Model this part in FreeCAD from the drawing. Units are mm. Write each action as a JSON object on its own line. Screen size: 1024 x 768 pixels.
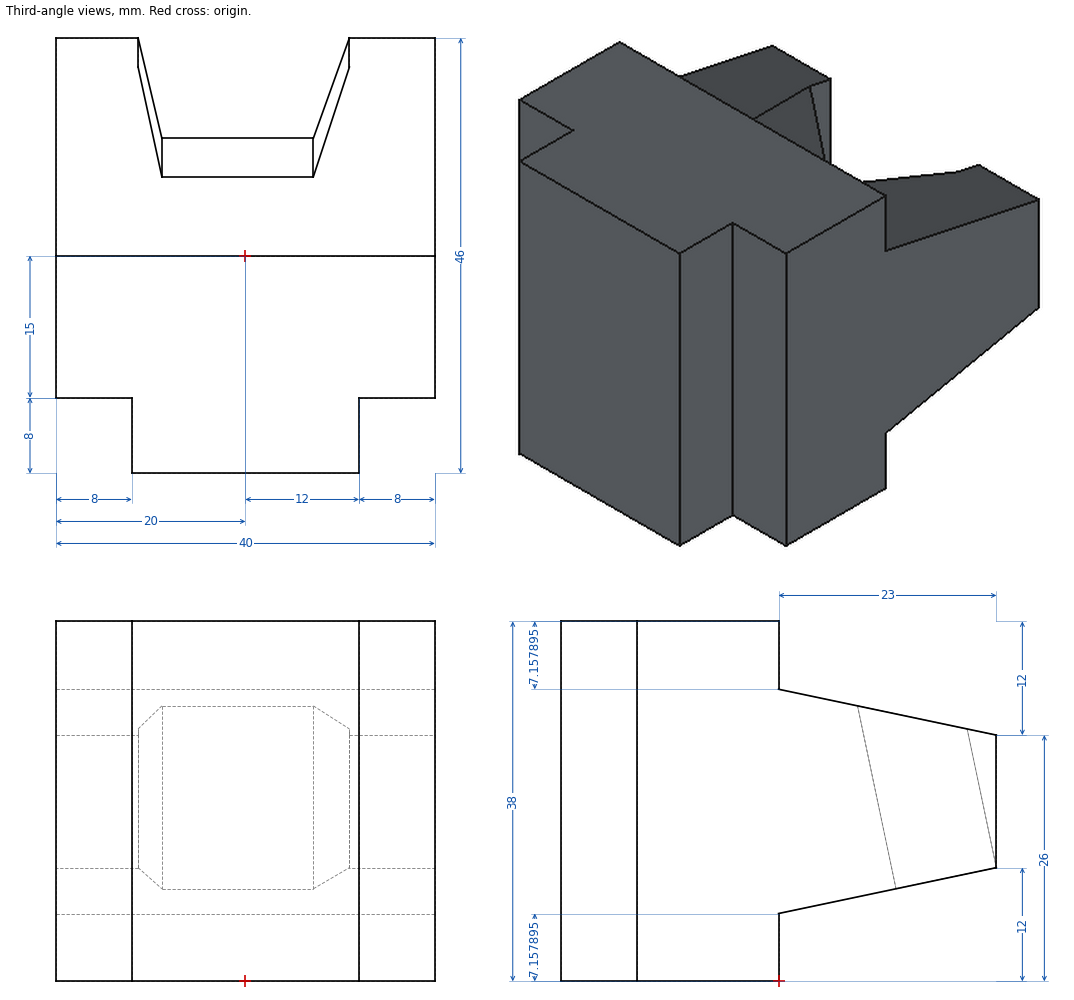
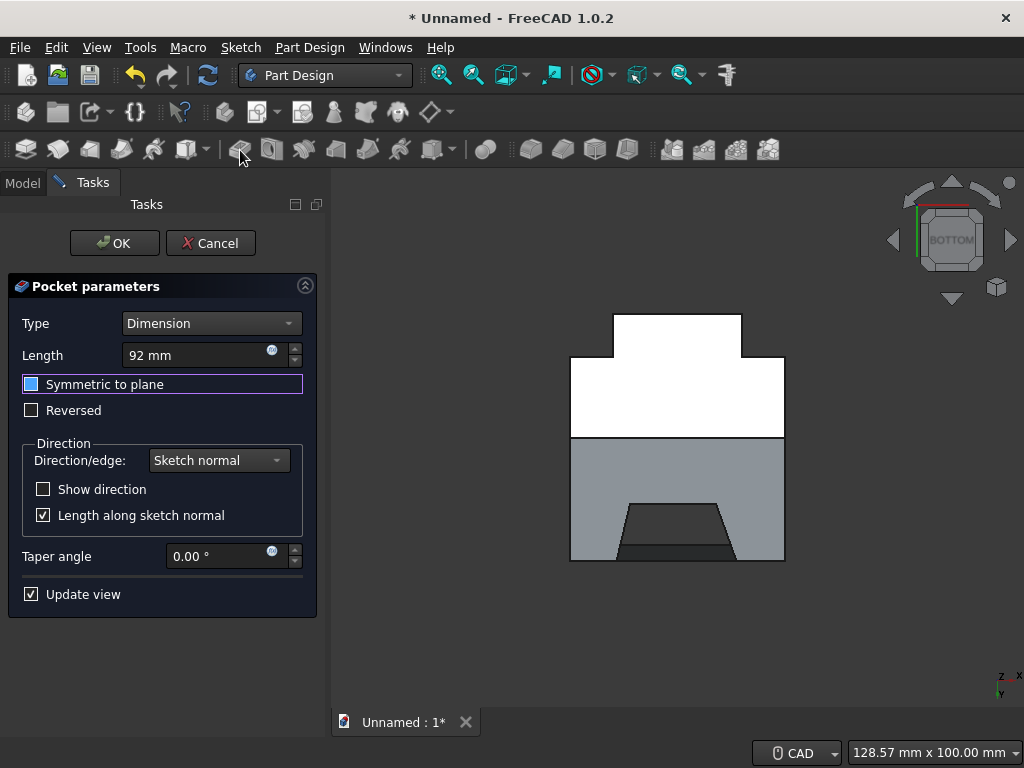
{"action": "left_click", "coordinate": [30, 384]}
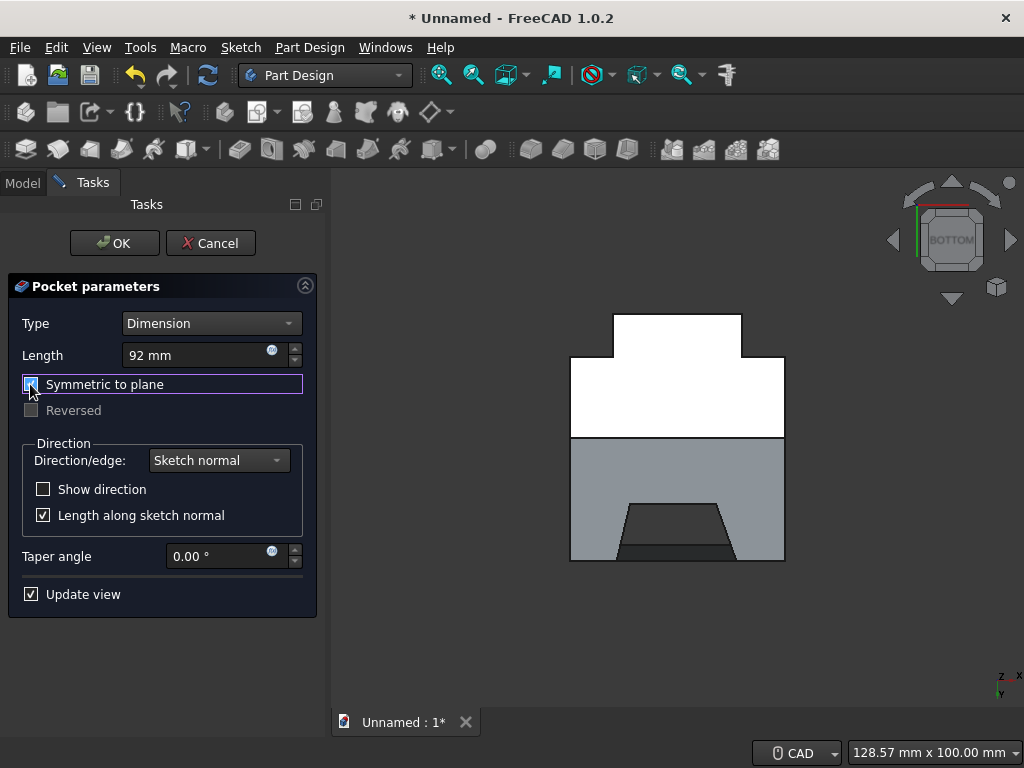
{"action": "left_click", "coordinate": [115, 243]}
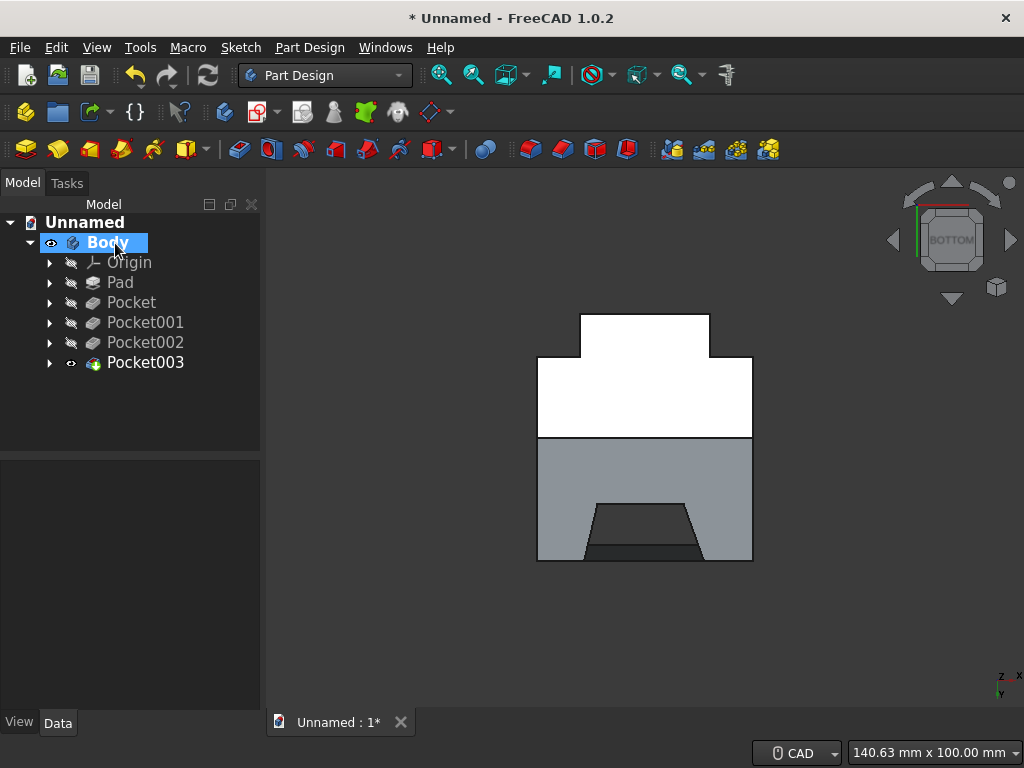
{"action": "left_click", "coordinate": [707, 481]}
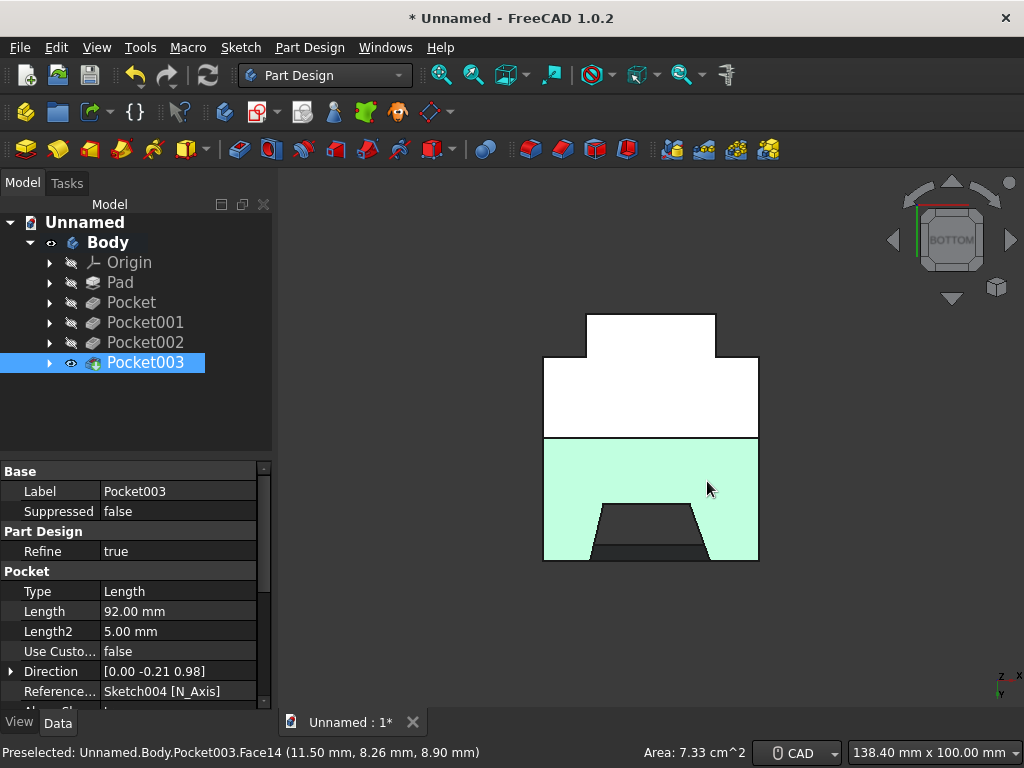
{"action": "left_click", "coordinate": [258, 112]}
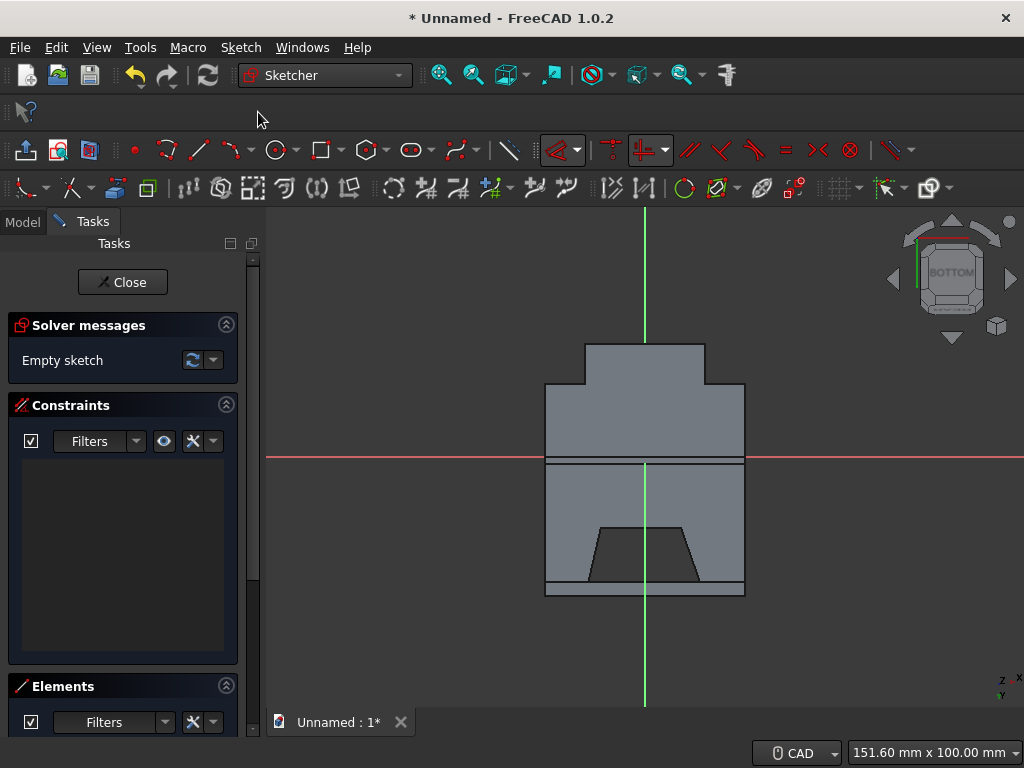
{"action": "left_click", "coordinate": [90, 150]}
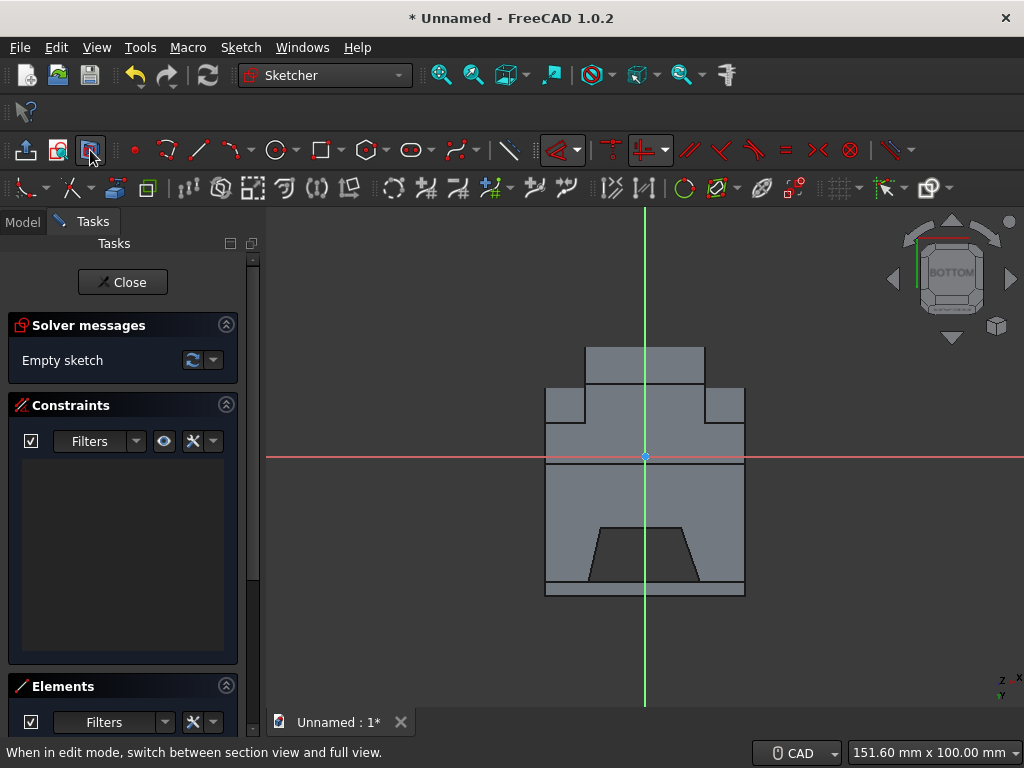
{"action": "scroll", "coordinate": [699, 592], "scroll_direction": "up", "scroll_amount": 4}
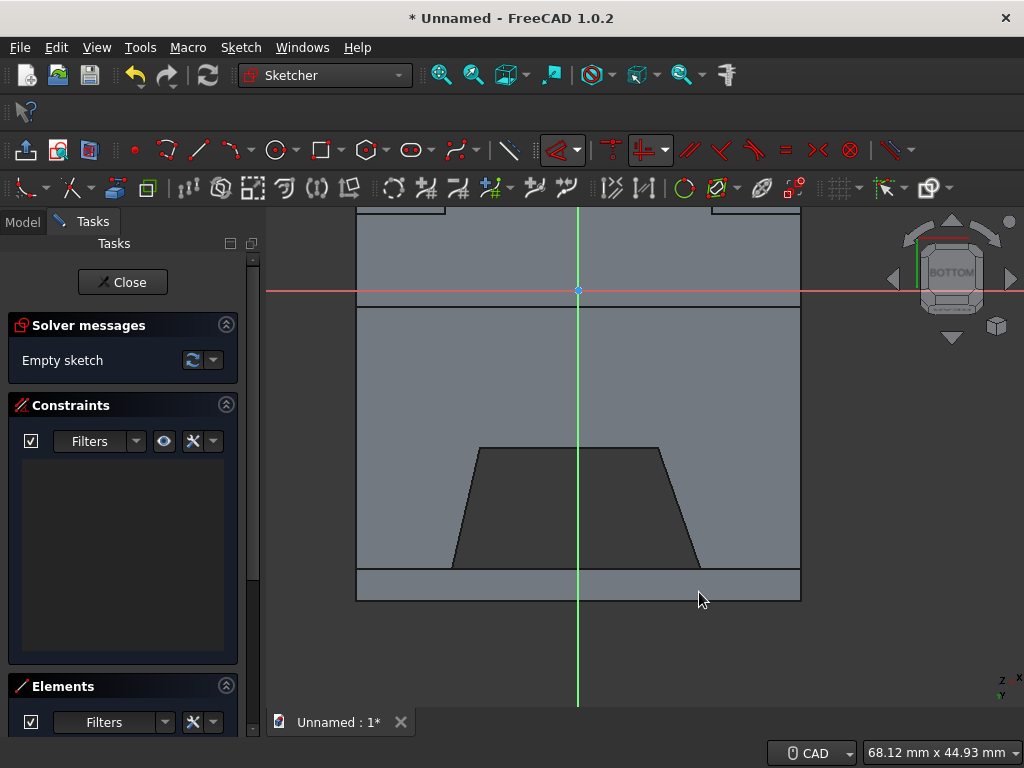
{"action": "left_click", "coordinate": [322, 150]}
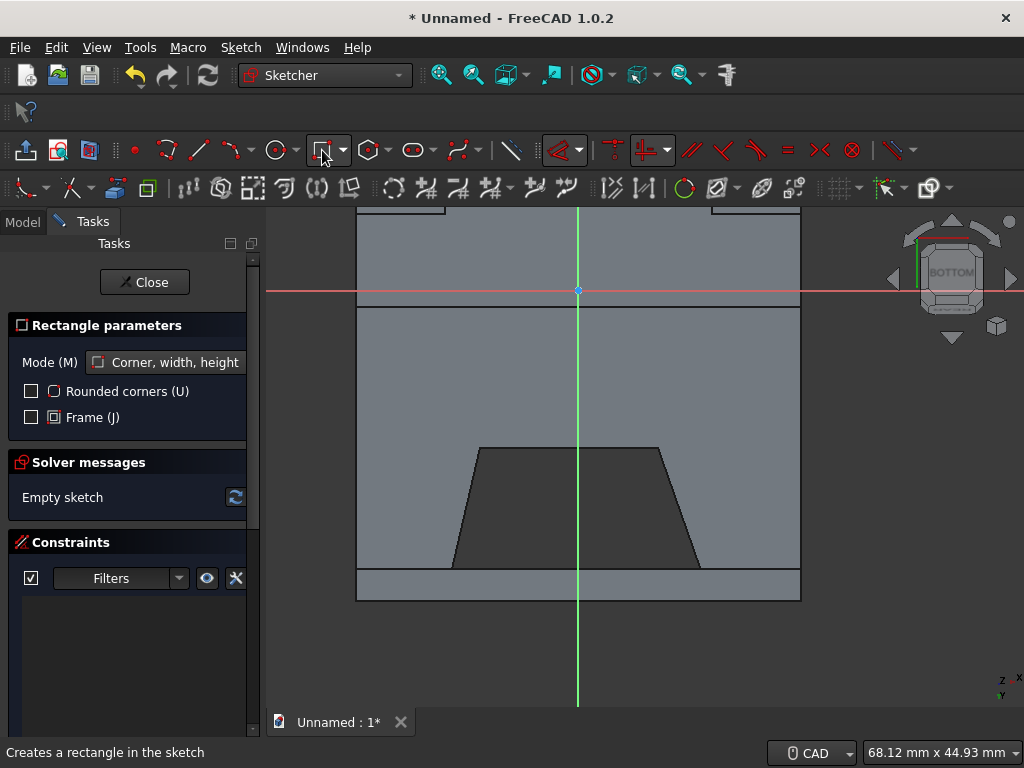
{"action": "left_click", "coordinate": [452, 569]}
{"action": "left_click", "coordinate": [700, 621]}
{"action": "key", "text": "Escape"}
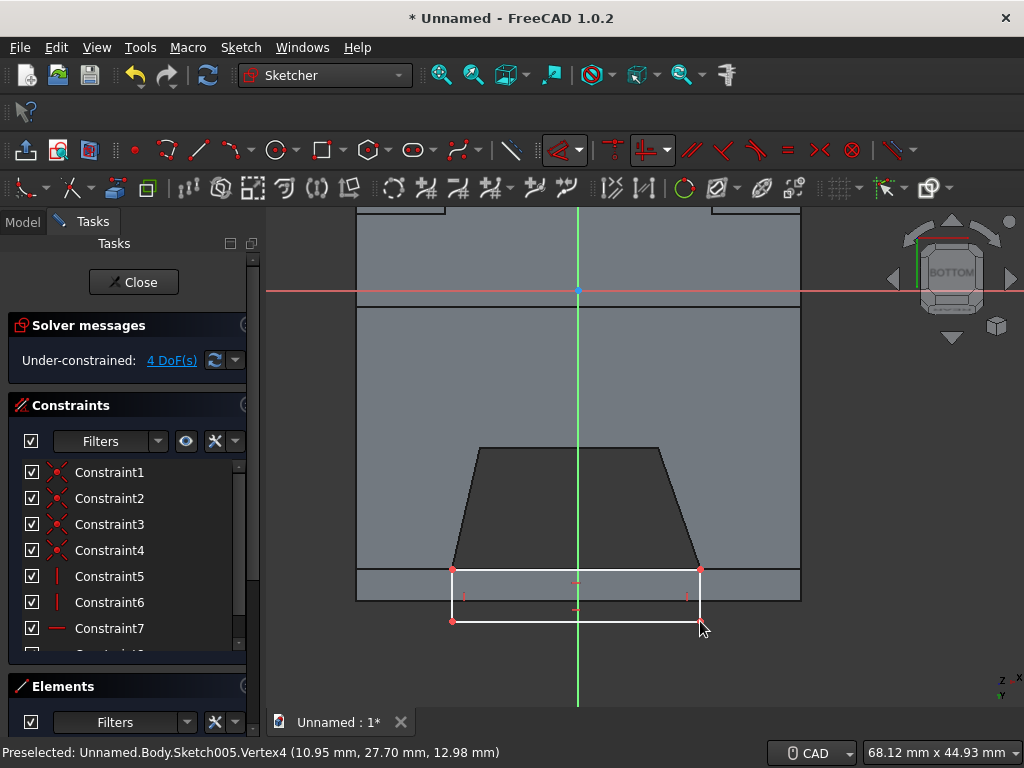
{"action": "left_click", "coordinate": [452, 586]}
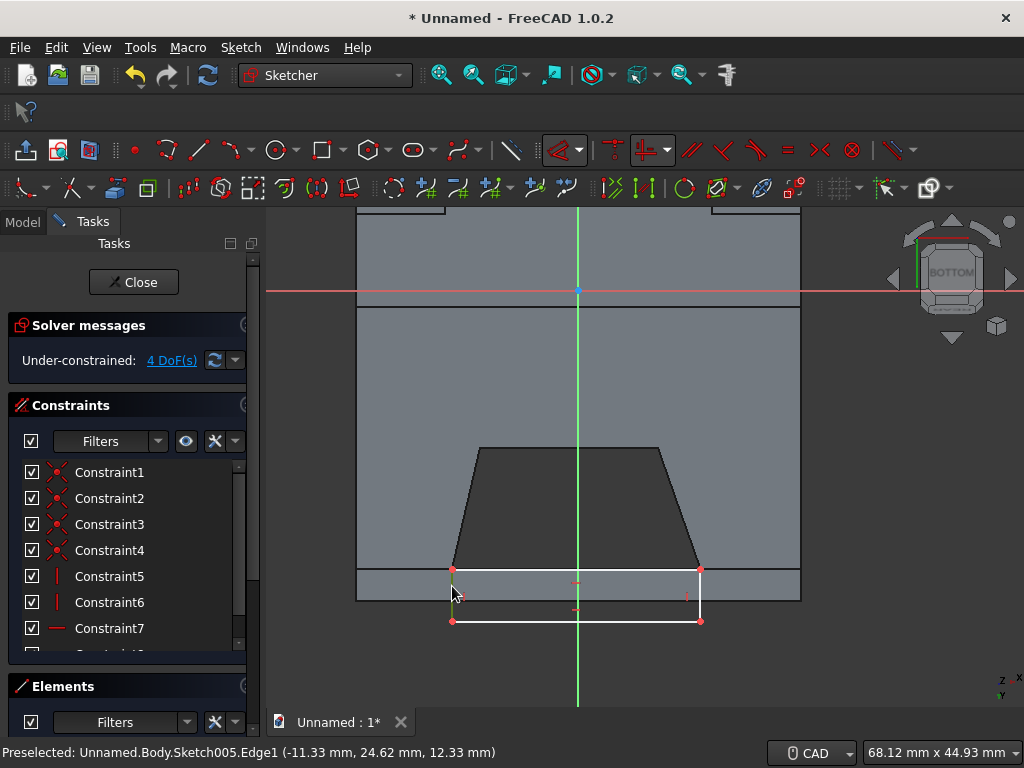
{"action": "left_click", "coordinate": [582, 150]}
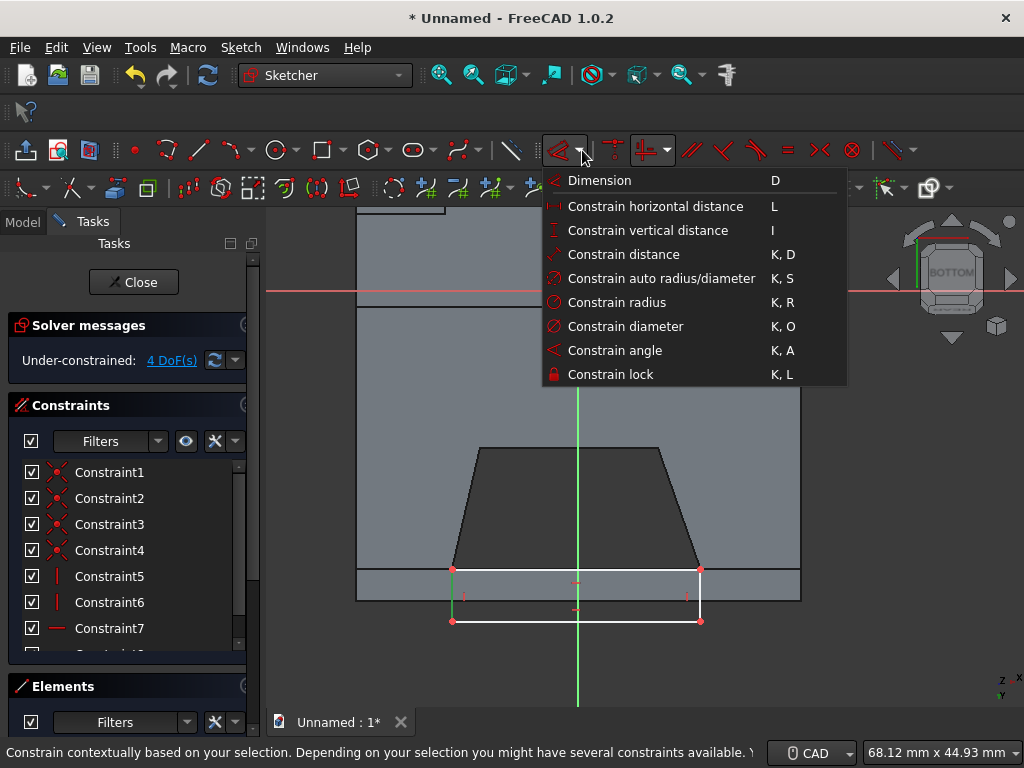
{"action": "left_click", "coordinate": [695, 230]}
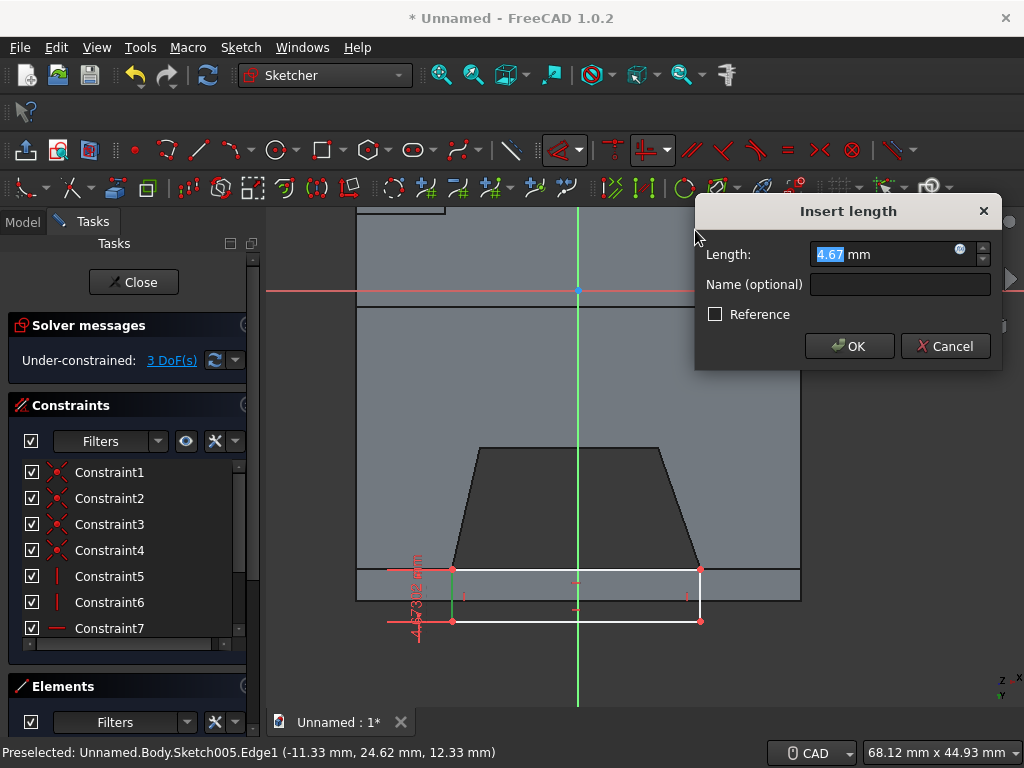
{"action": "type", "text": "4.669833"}
{"action": "key", "text": "Return"}